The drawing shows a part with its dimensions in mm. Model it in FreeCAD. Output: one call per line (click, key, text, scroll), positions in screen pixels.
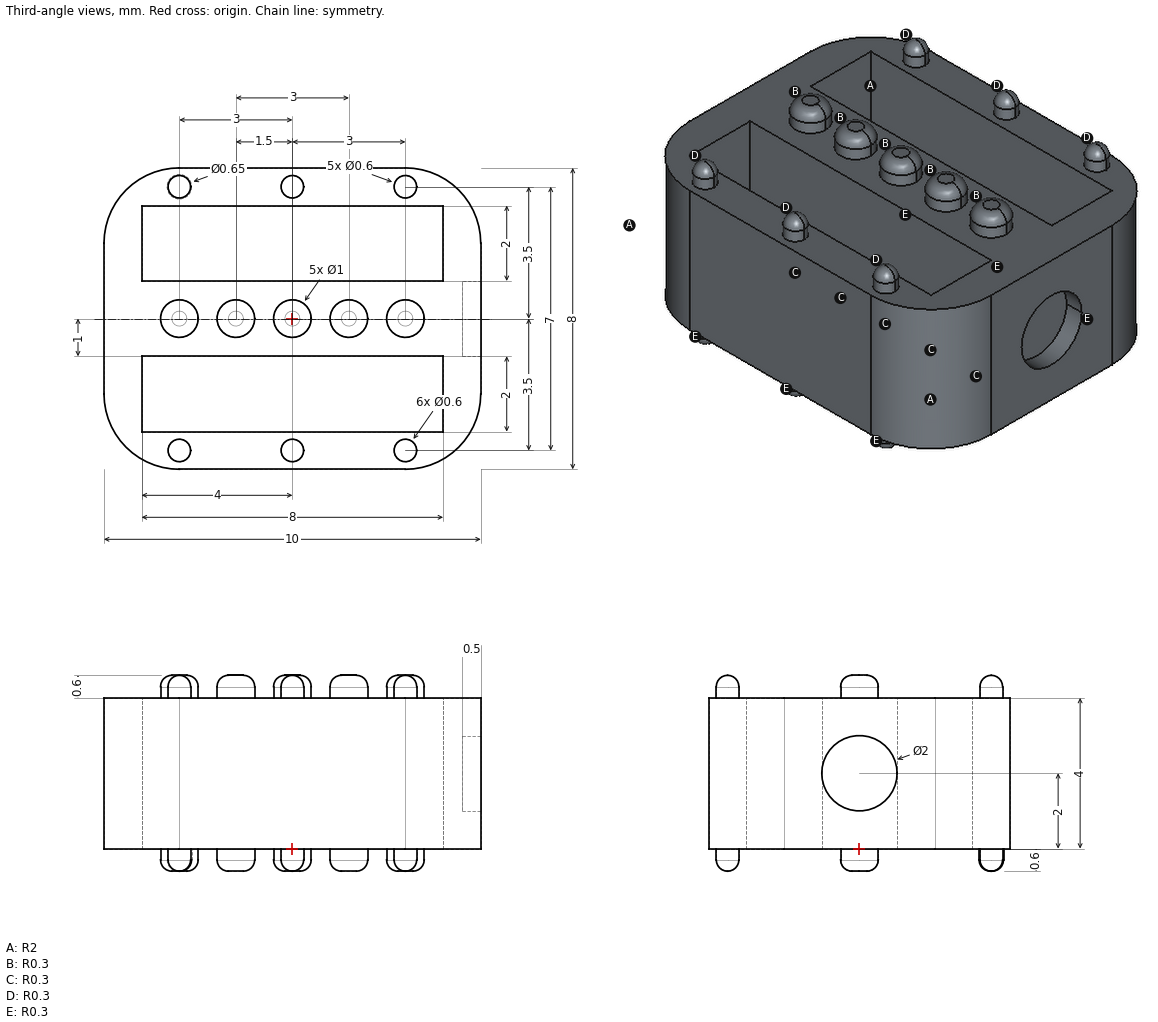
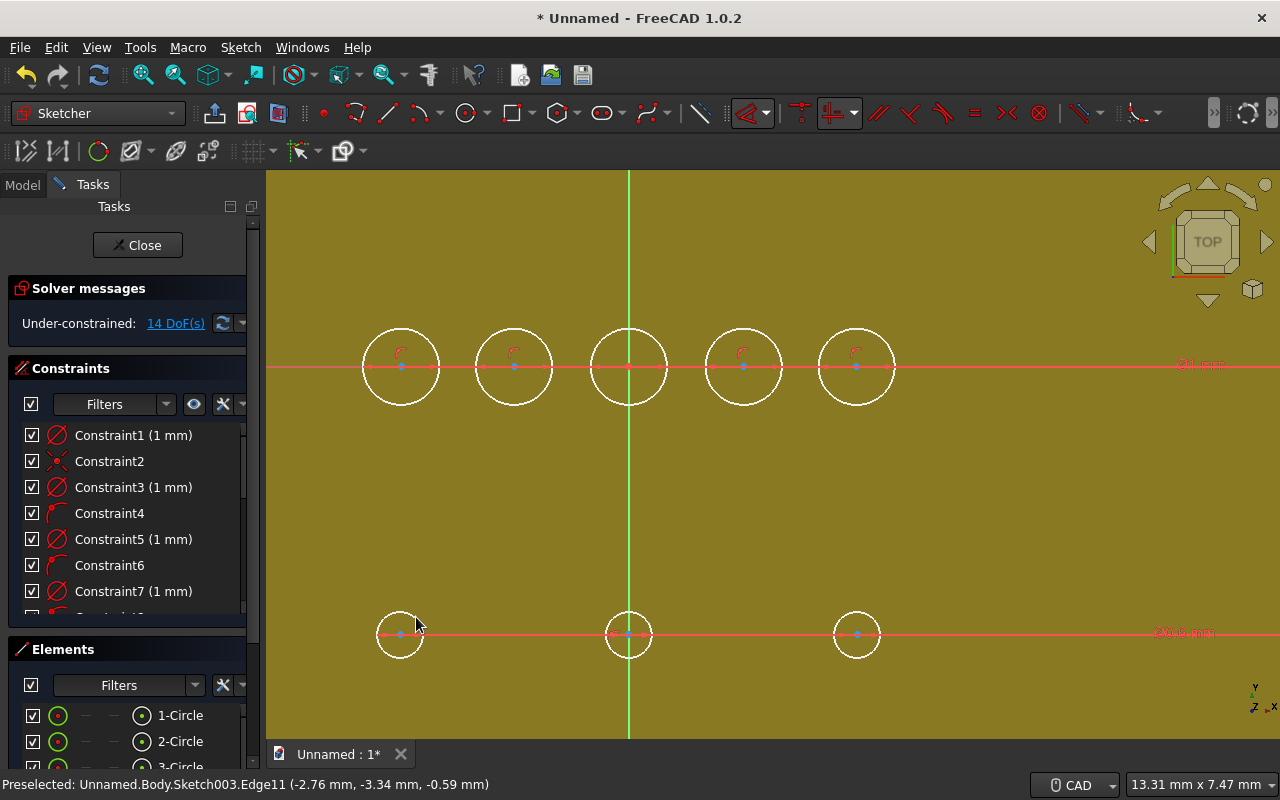
click(857, 367)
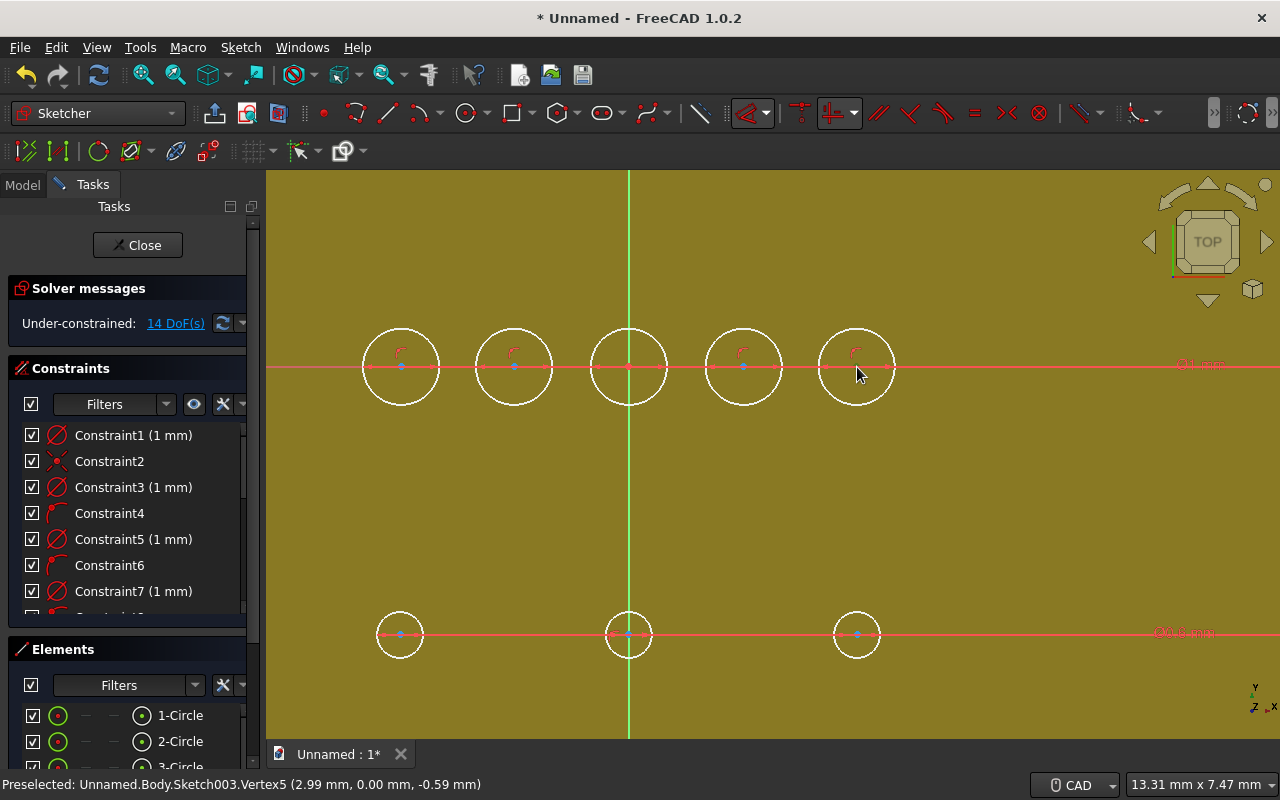
scroll(858, 635, down, 2)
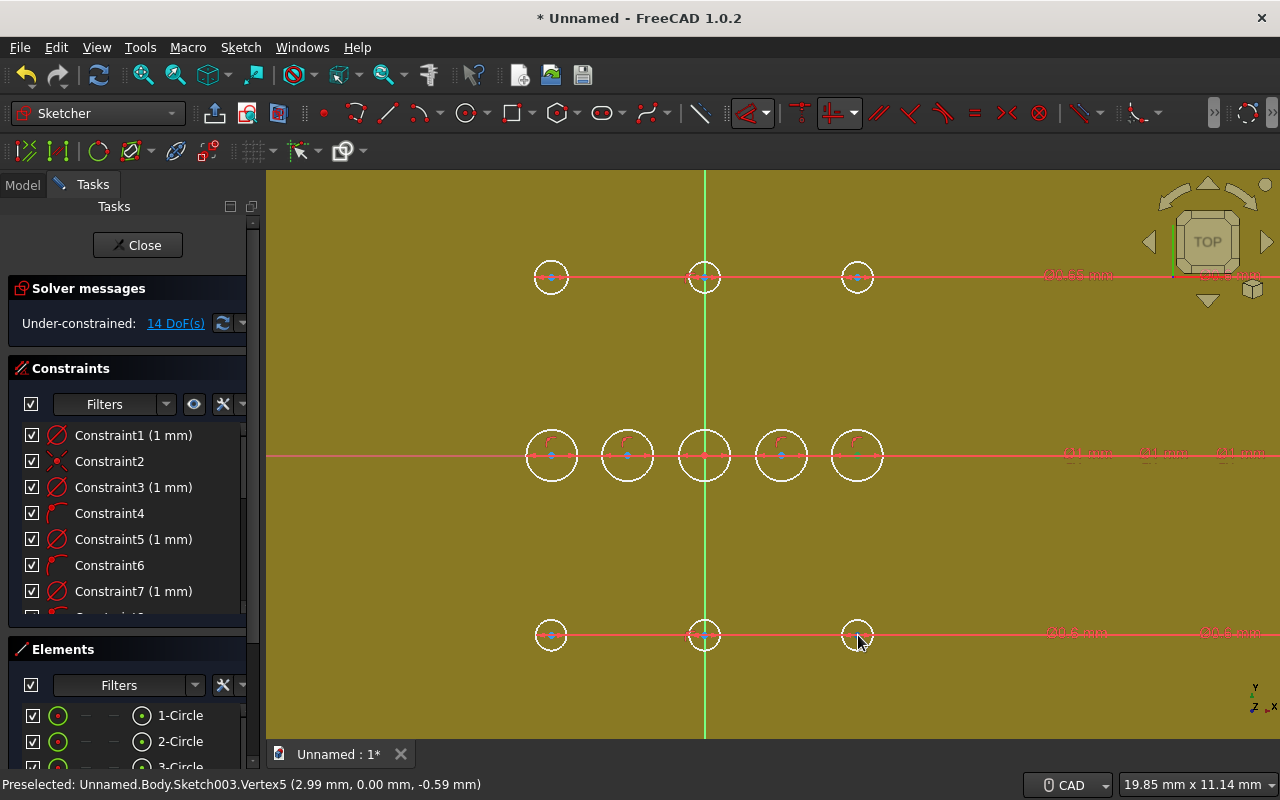
click(858, 277)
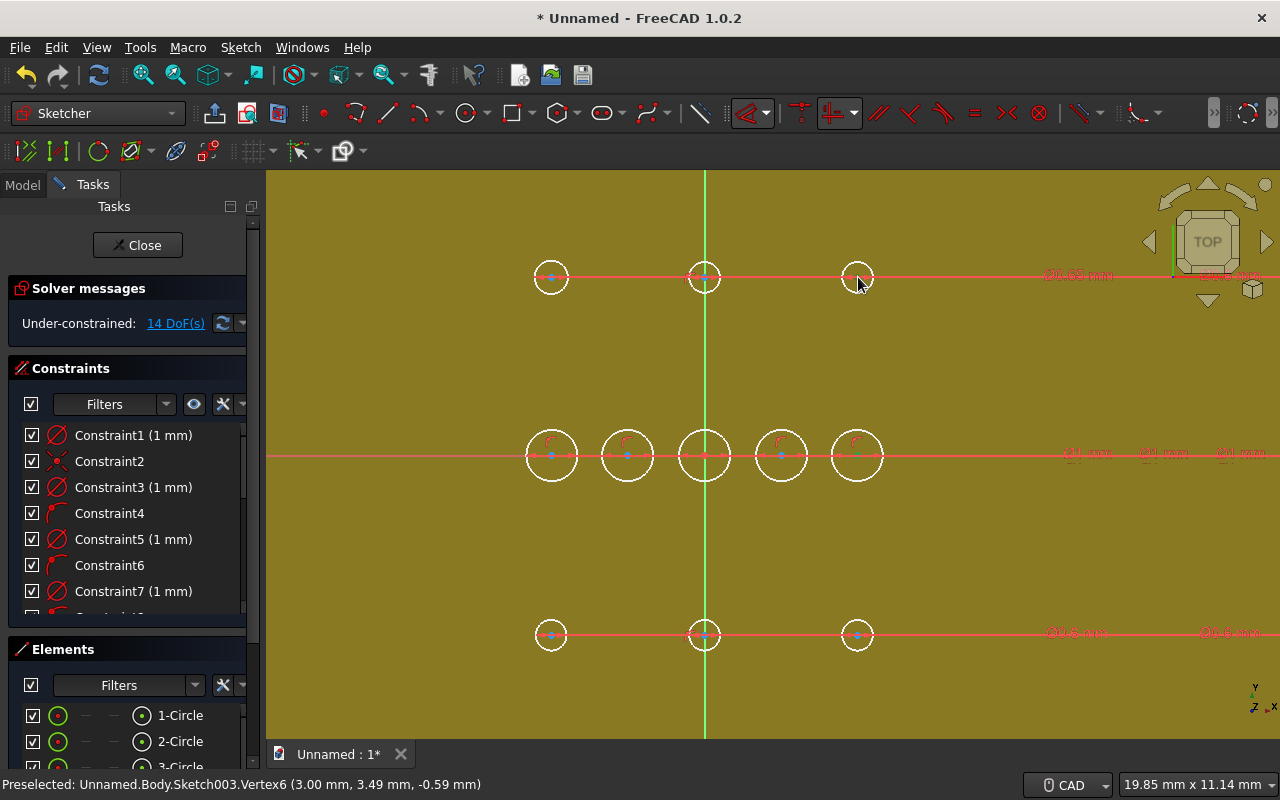
click(856, 114)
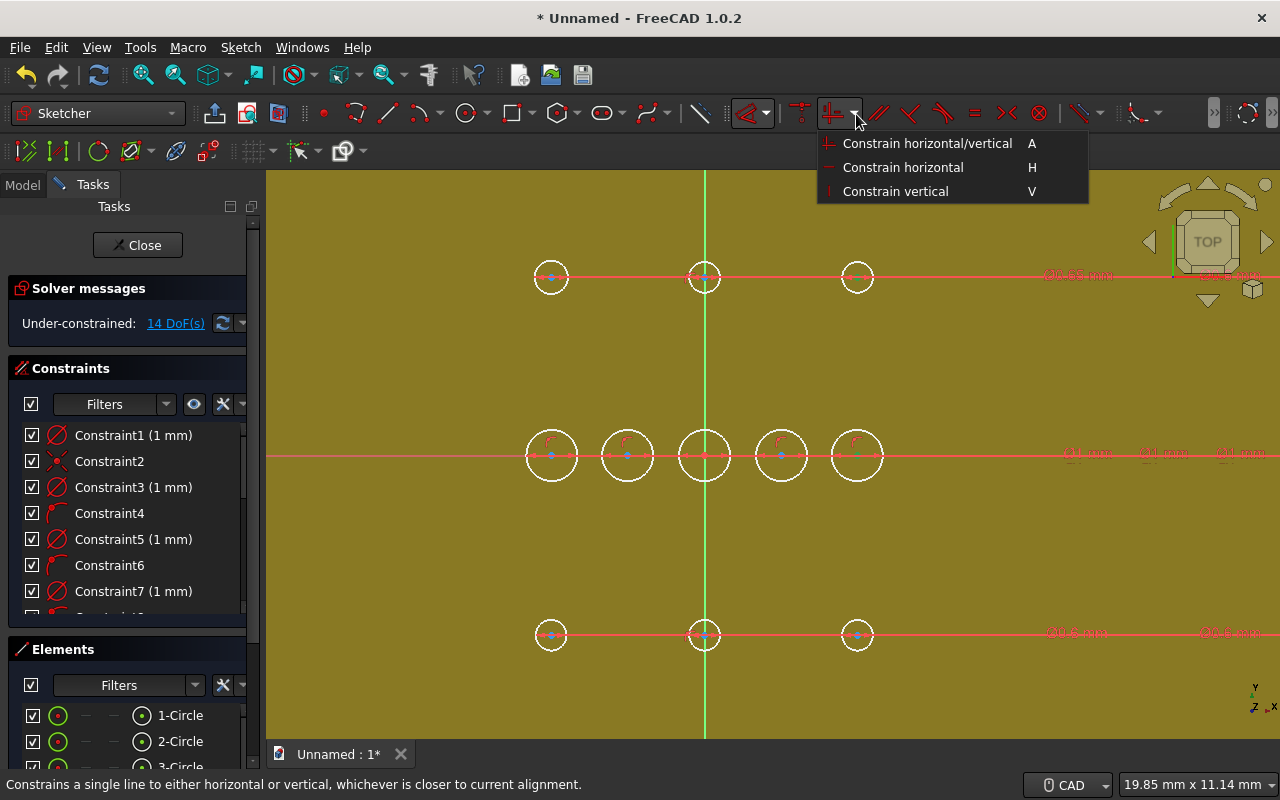
click(953, 191)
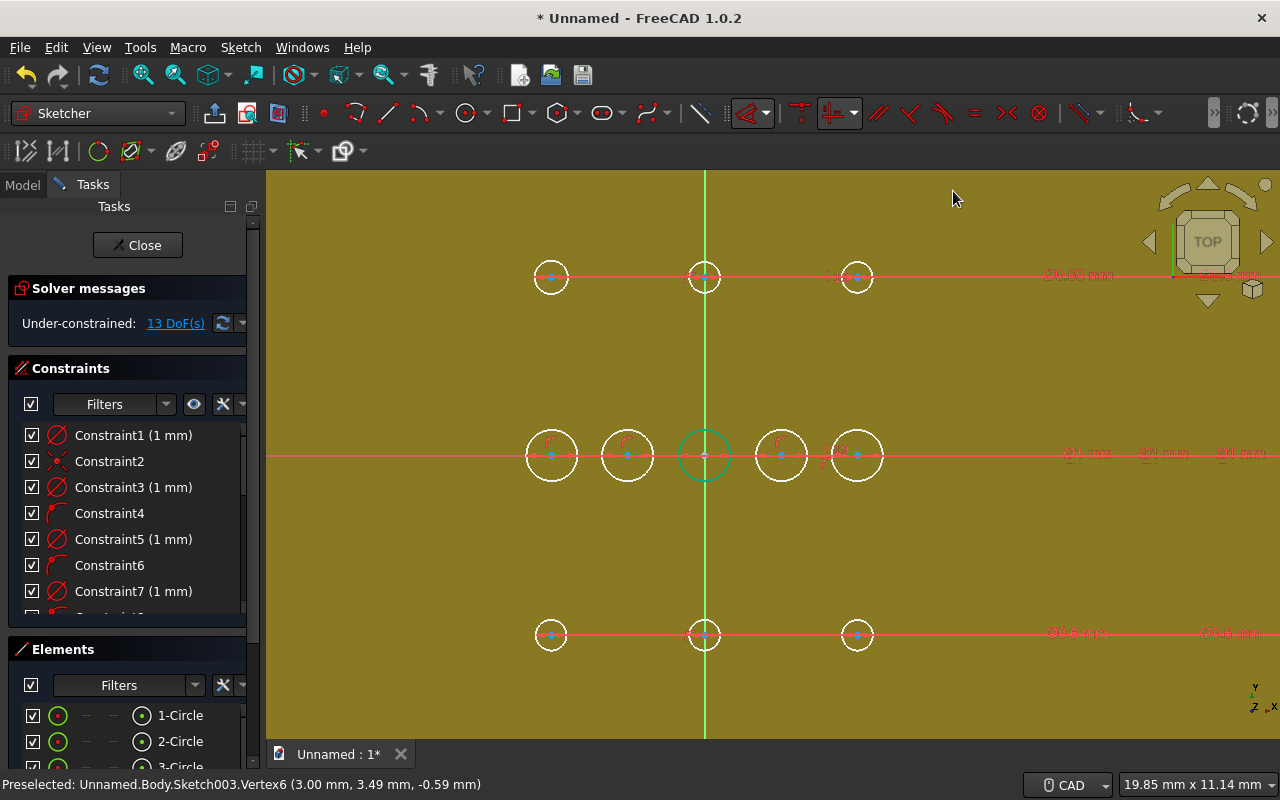
click(857, 277)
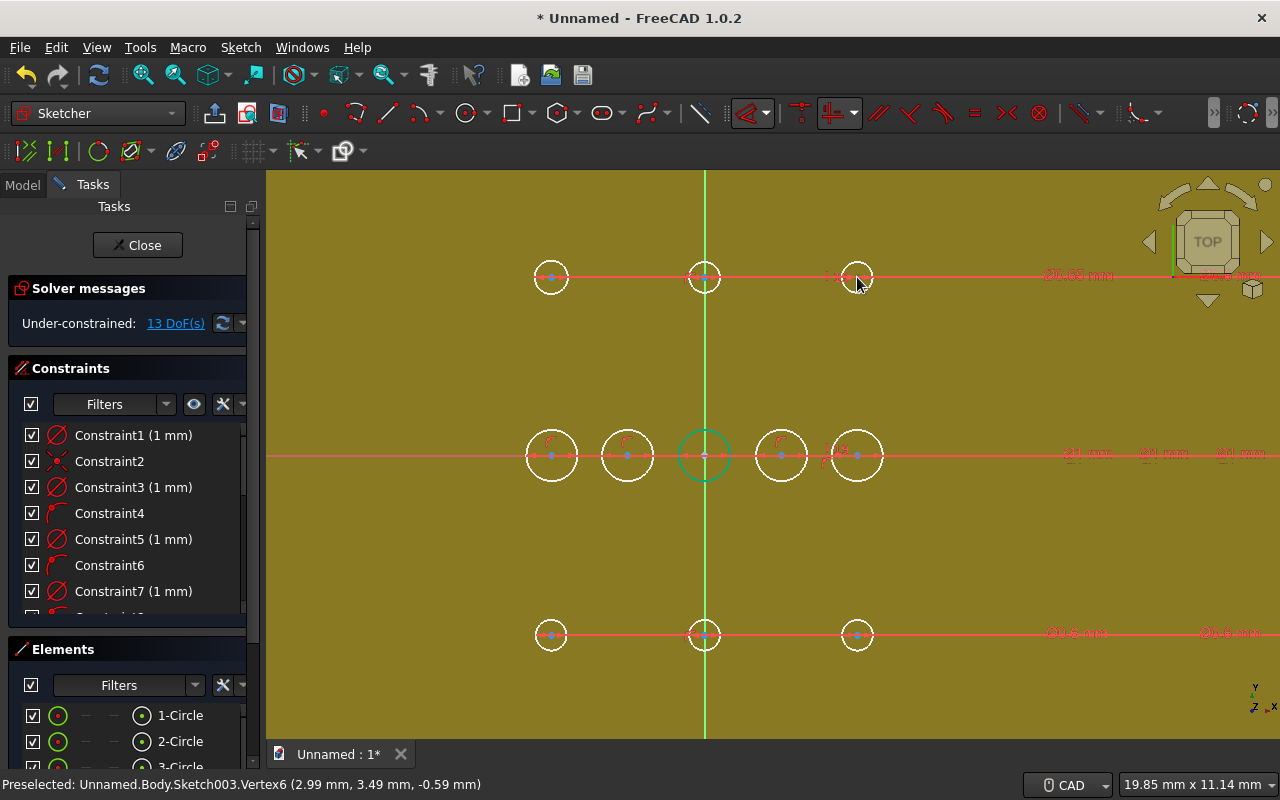
click(705, 277)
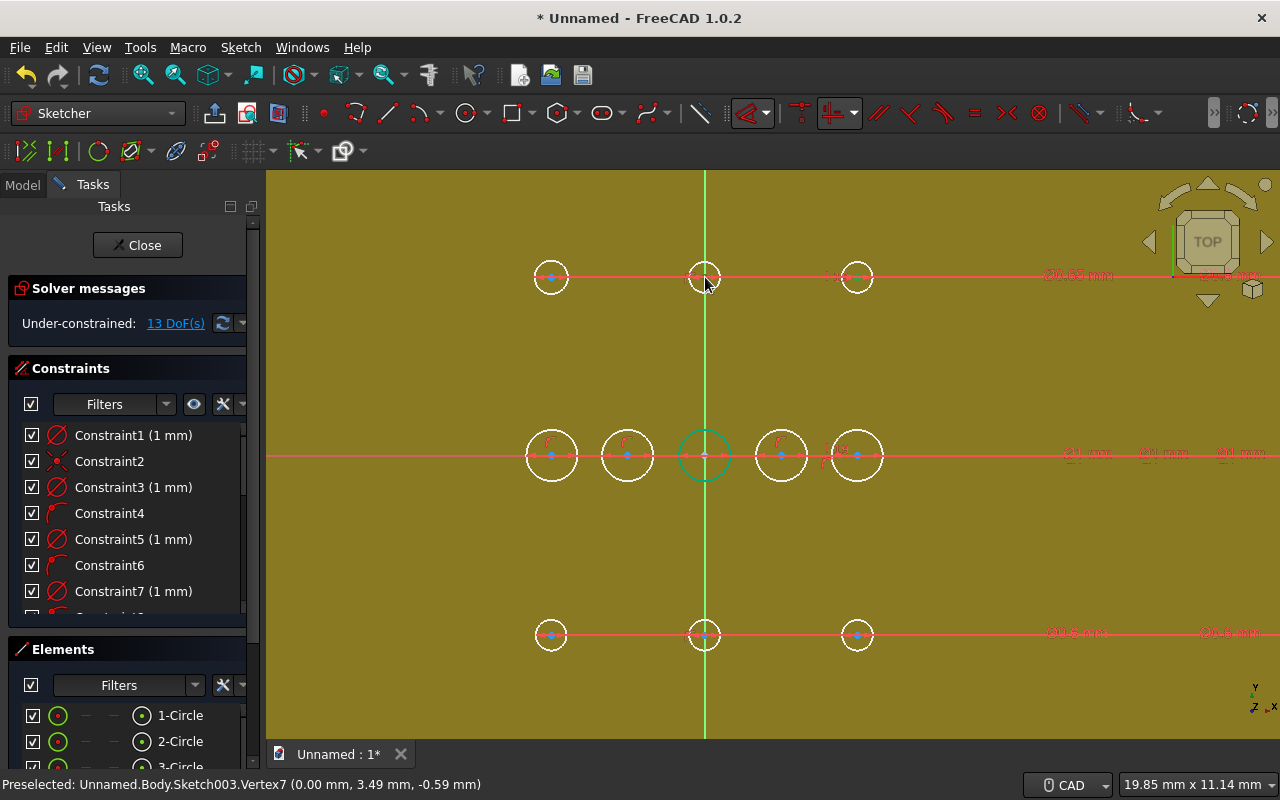
click(856, 114)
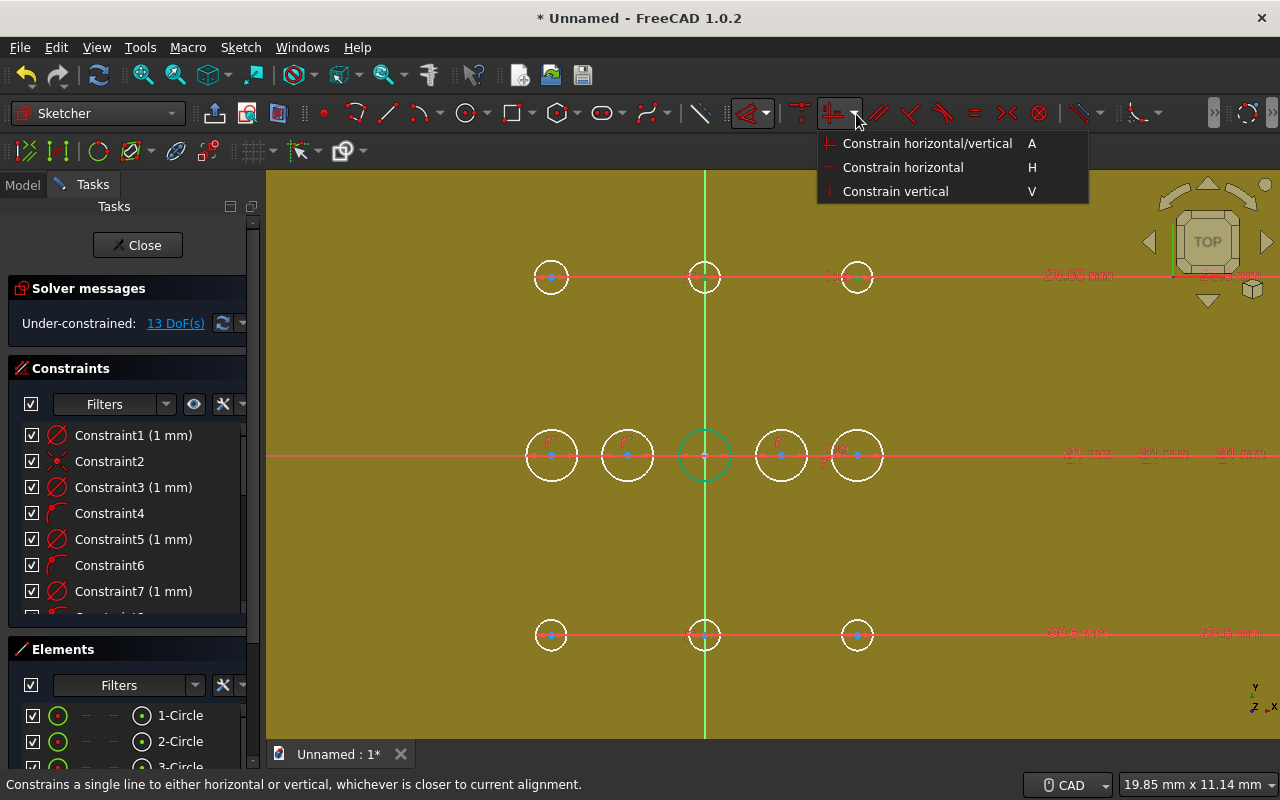
click(953, 167)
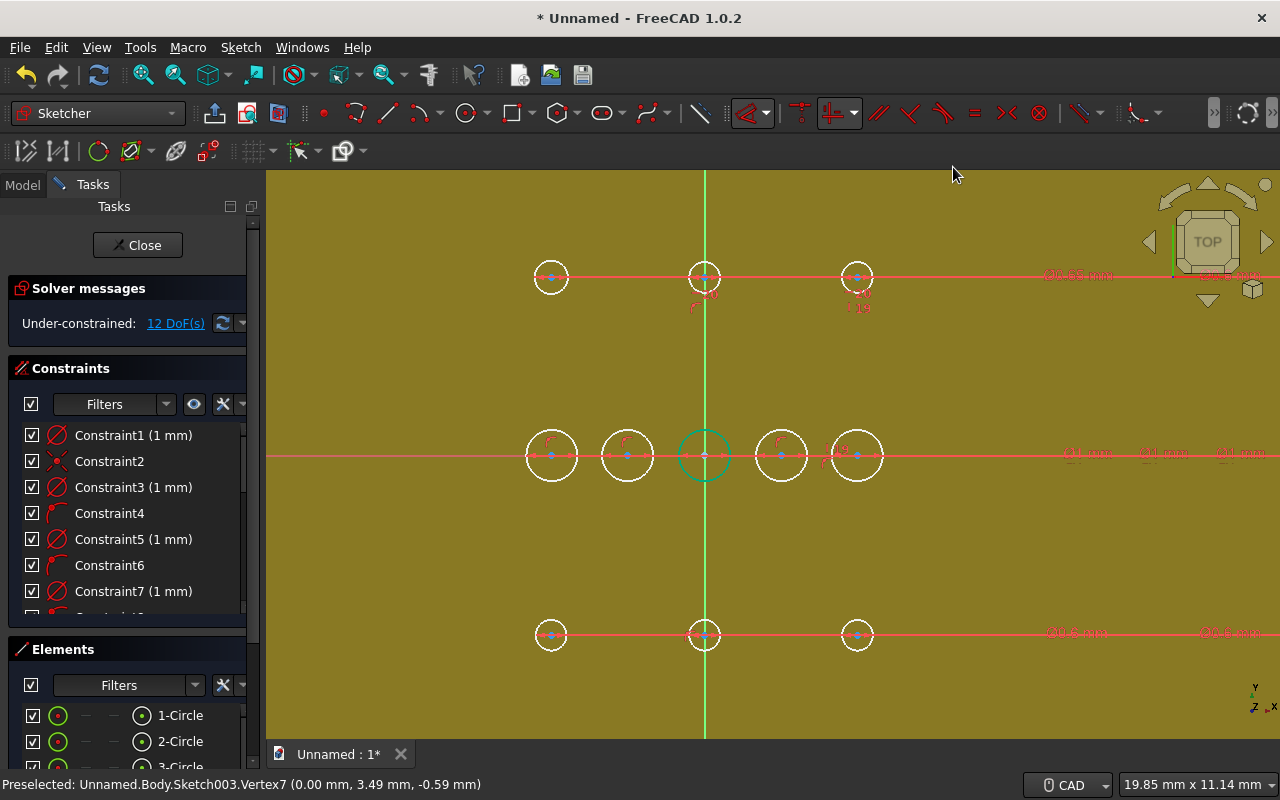
click(552, 456)